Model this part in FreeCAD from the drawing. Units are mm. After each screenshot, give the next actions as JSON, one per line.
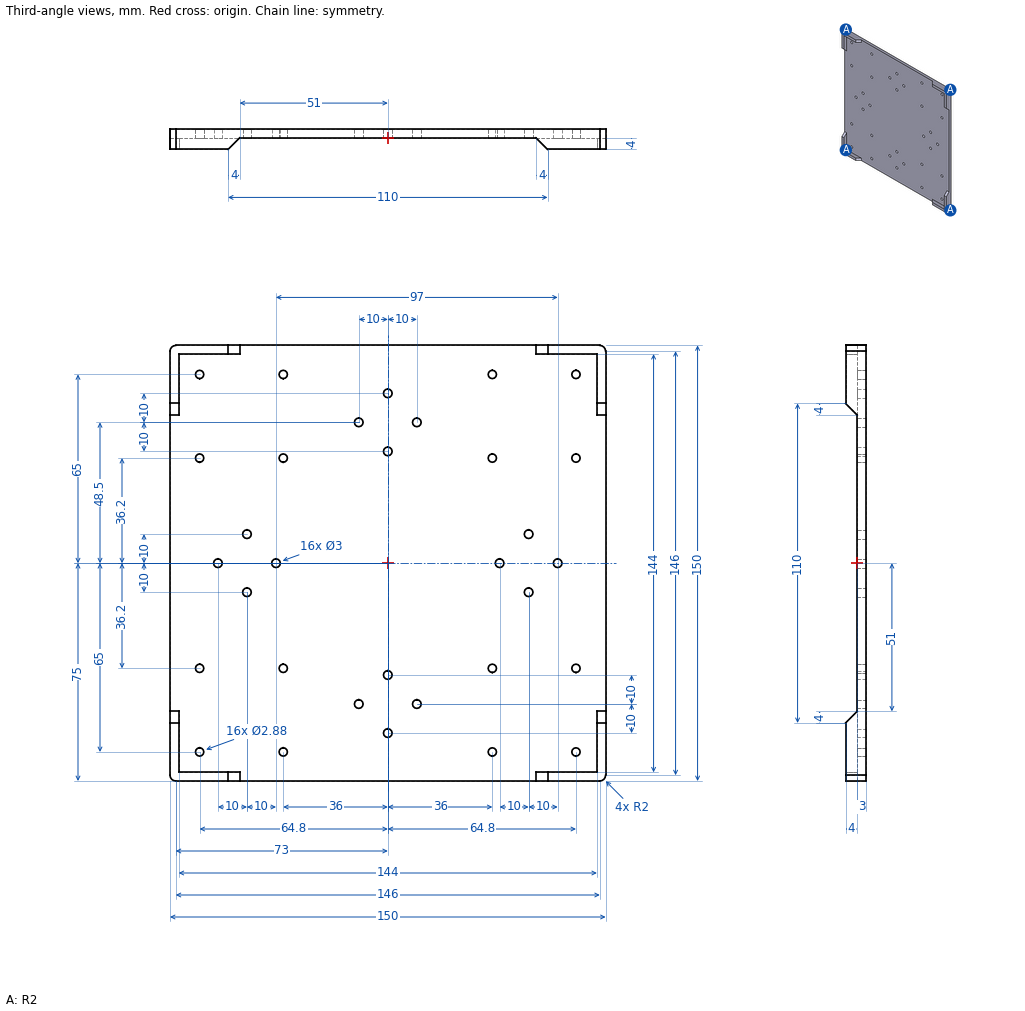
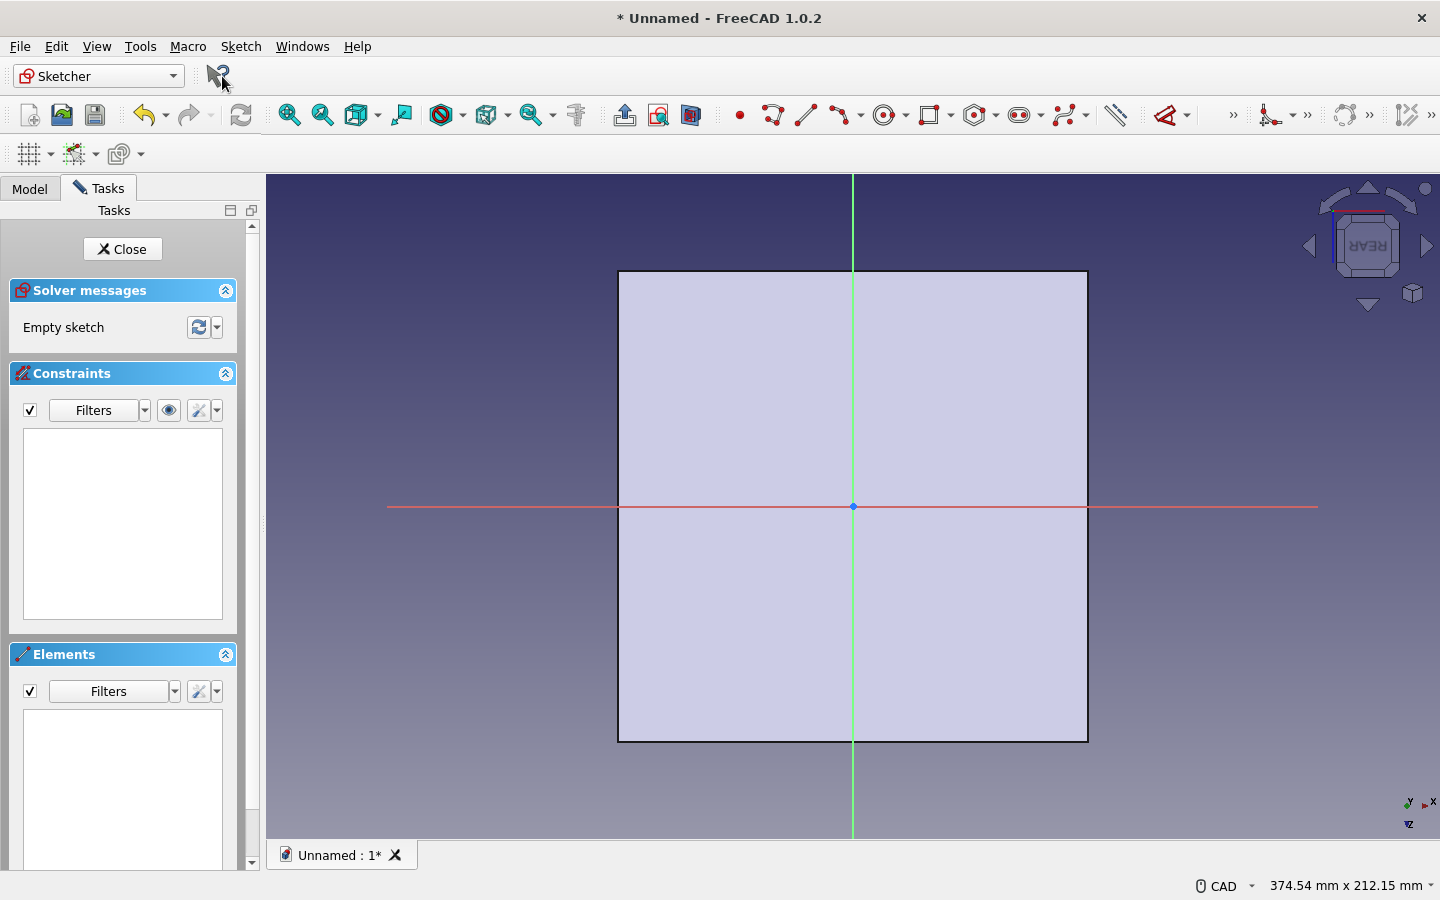
{"action": "left_click", "coordinate": [884, 116]}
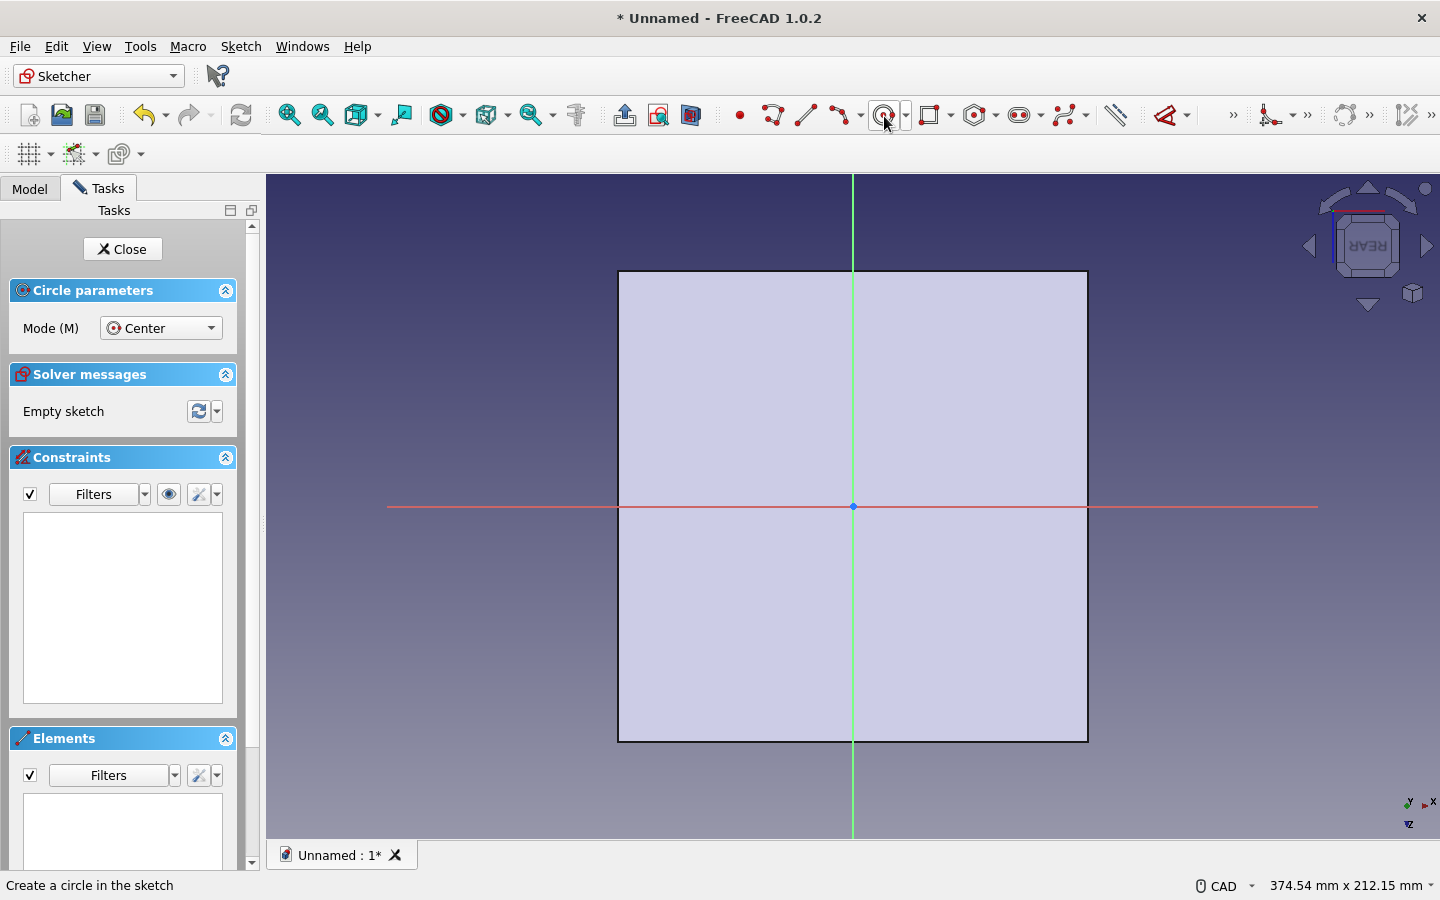
{"action": "scroll", "coordinate": [650, 303], "scroll_direction": "up", "scroll_amount": 9}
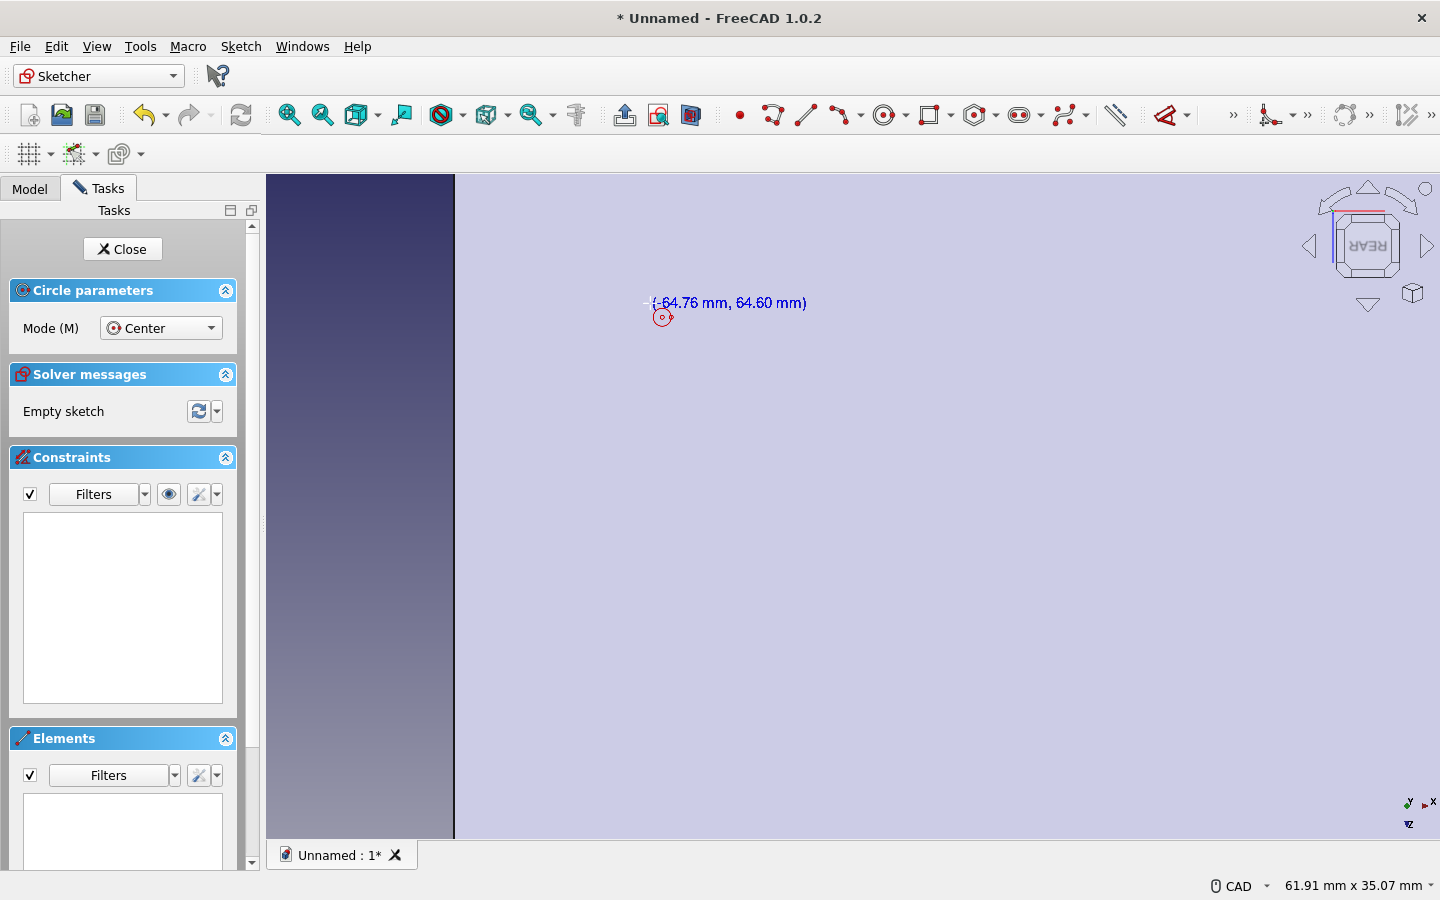
{"action": "scroll", "coordinate": [568, 303], "scroll_direction": "down", "scroll_amount": 9}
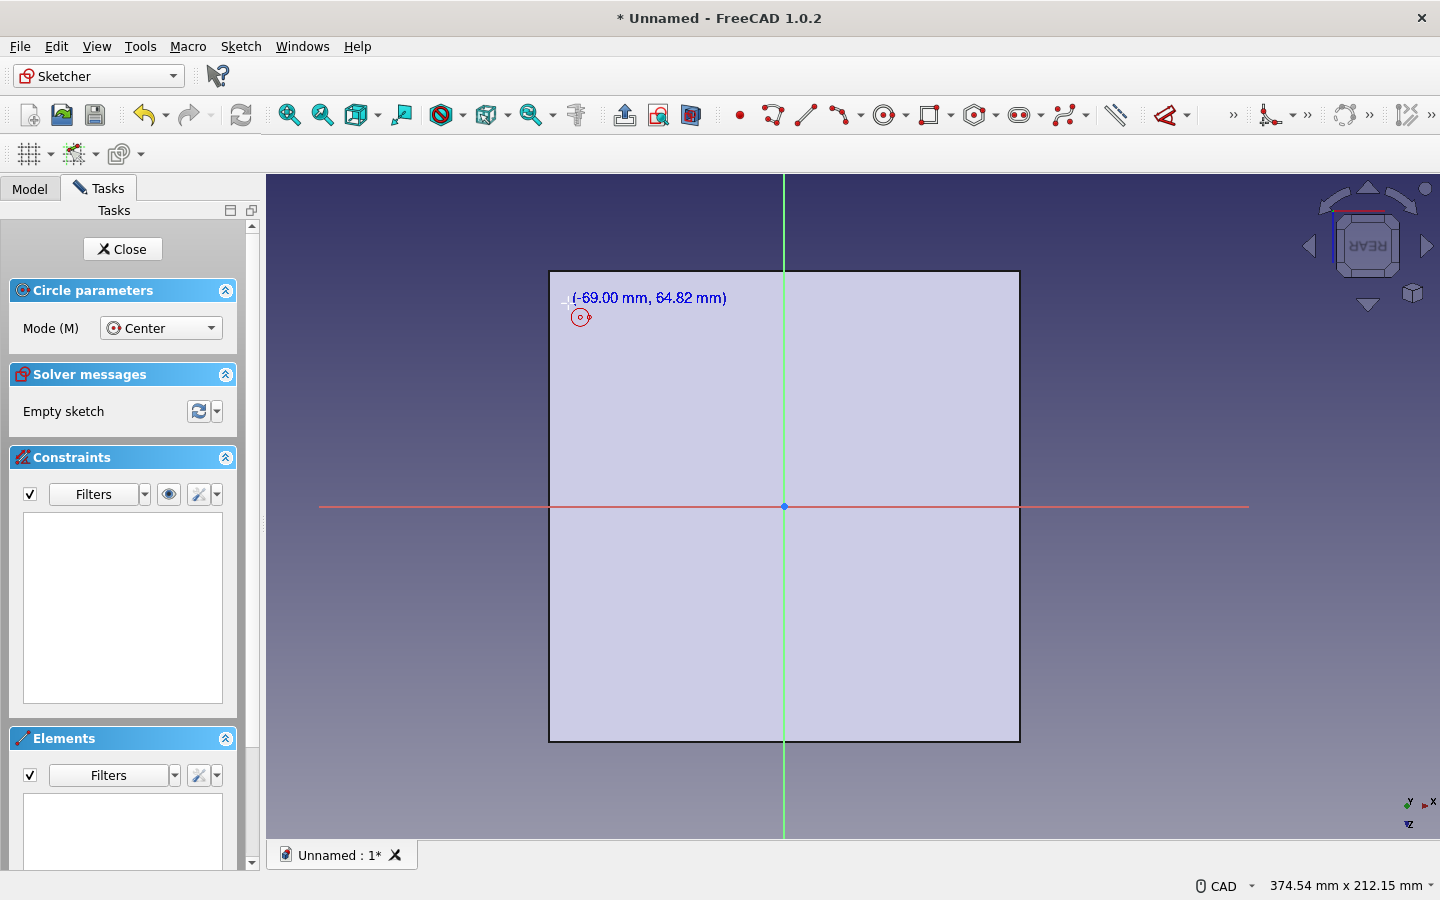
{"action": "left_click", "coordinate": [581, 303]}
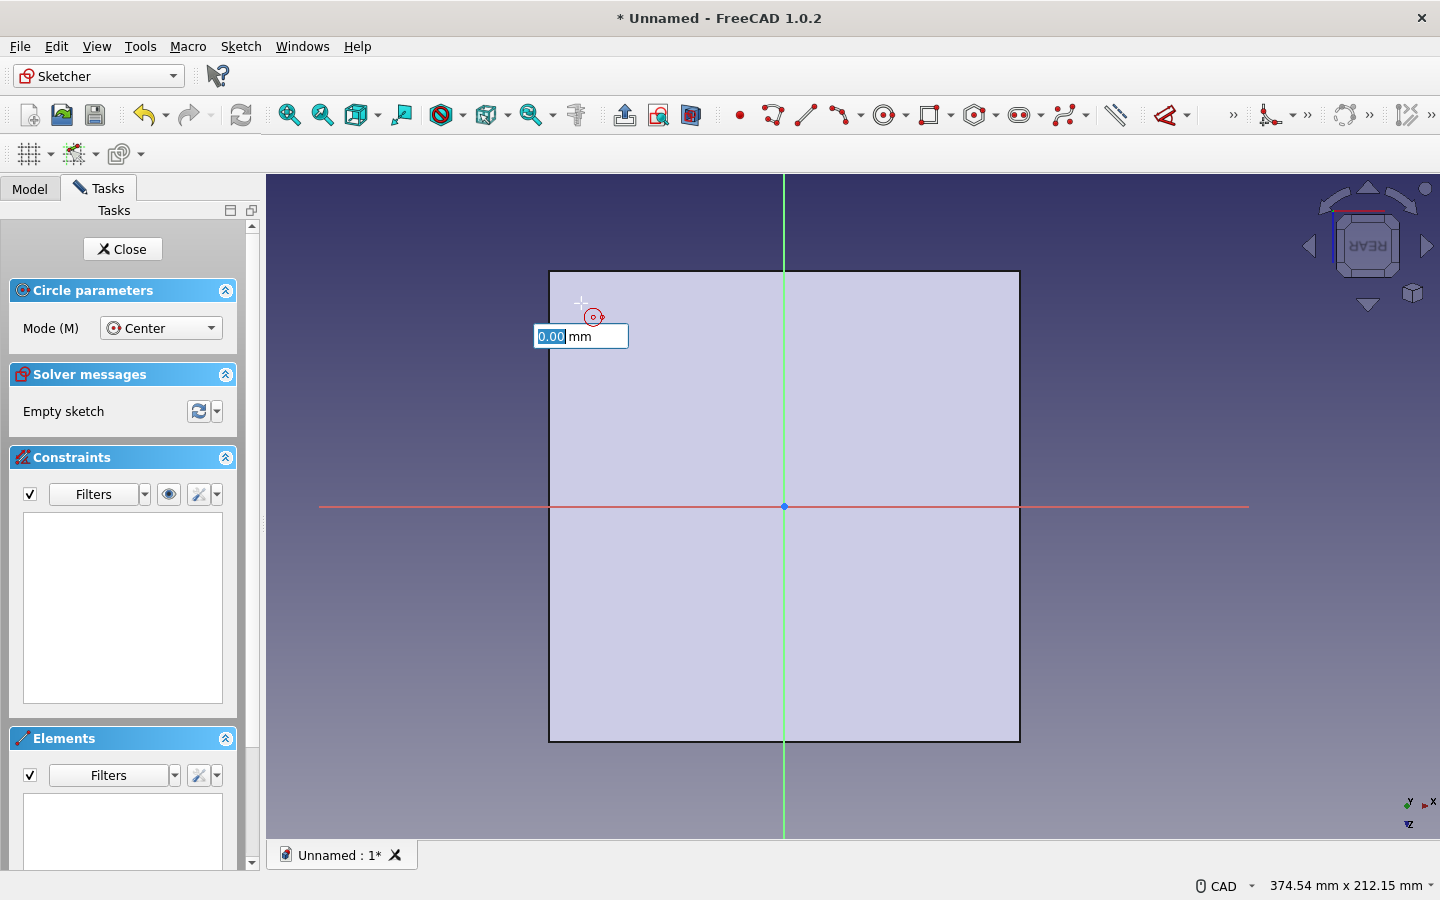
{"action": "scroll", "coordinate": [585, 300], "scroll_direction": "up", "scroll_amount": 7}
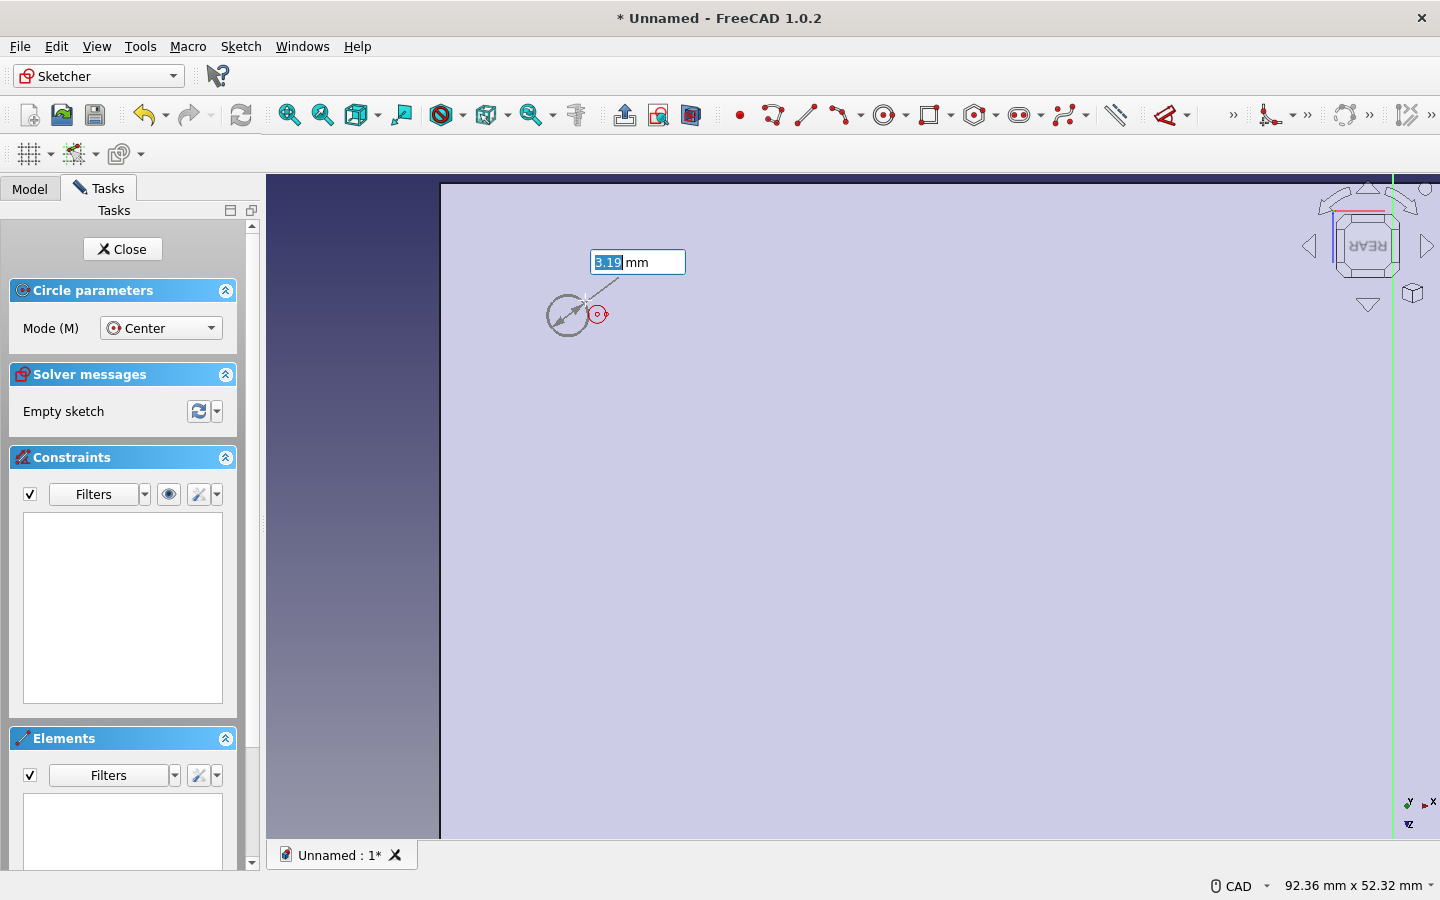
{"action": "left_click", "coordinate": [582, 298]}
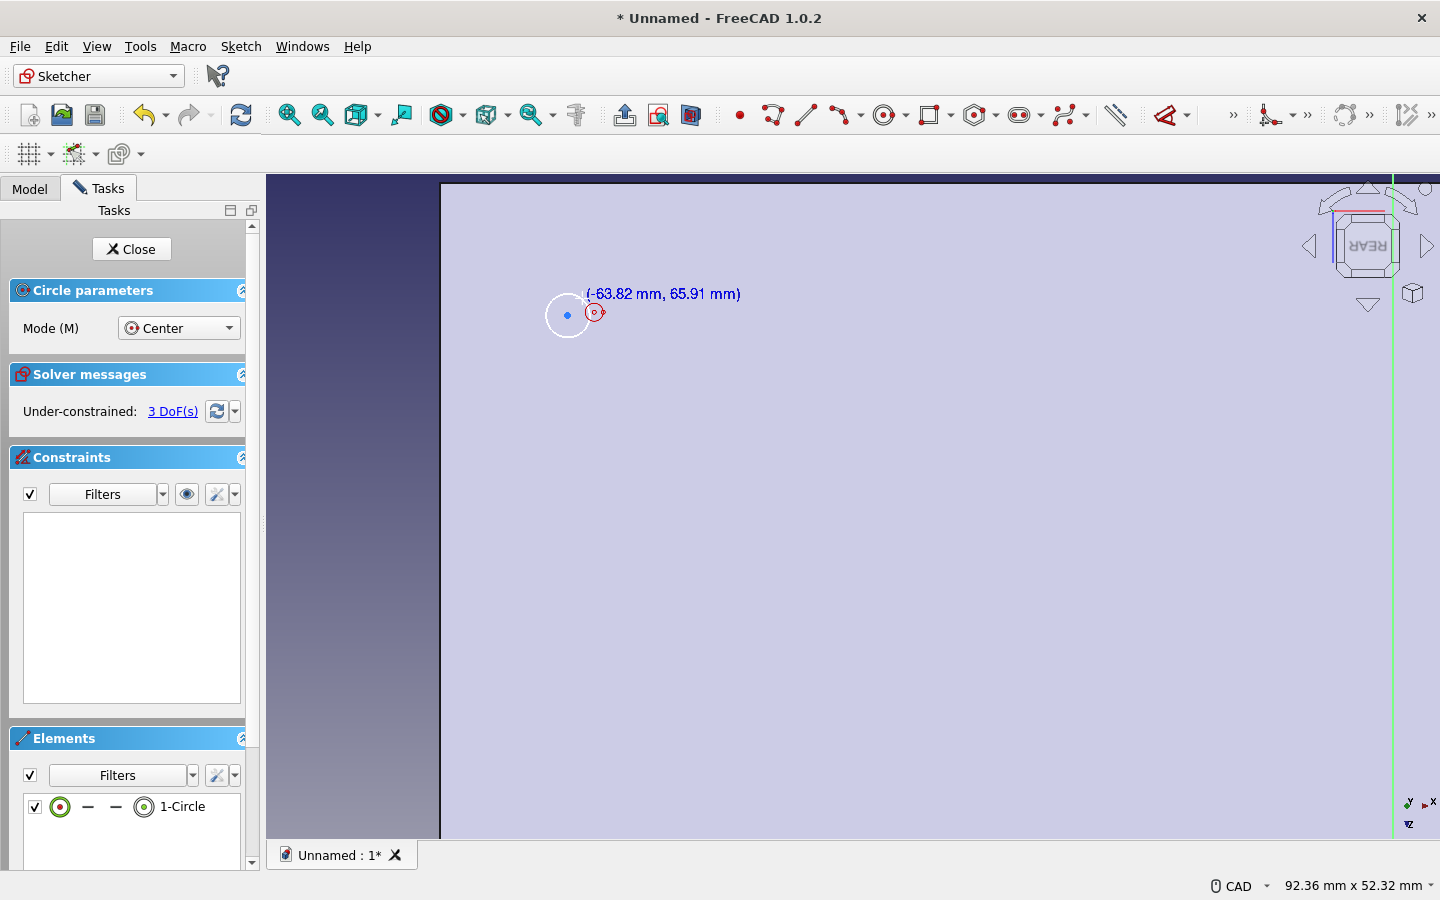
{"action": "scroll", "coordinate": [936, 311], "scroll_direction": "up", "scroll_amount": 2}